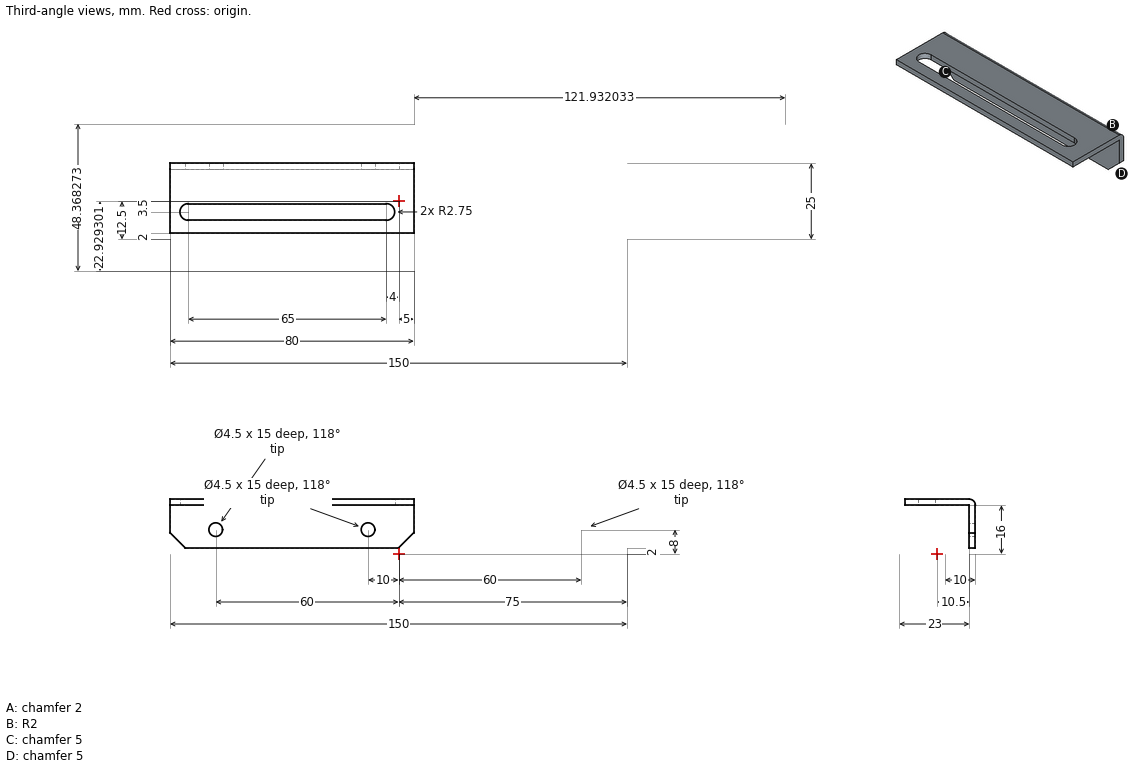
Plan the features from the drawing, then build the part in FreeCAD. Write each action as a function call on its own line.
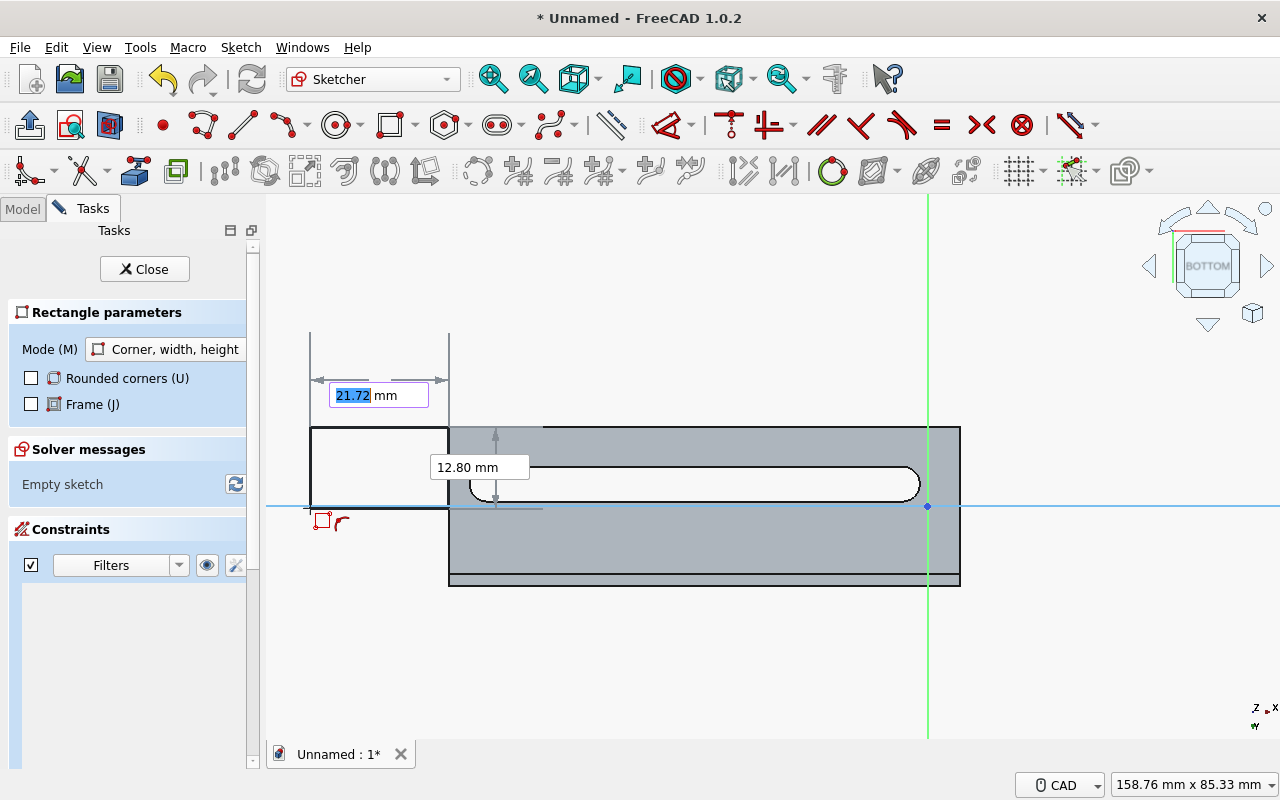
click(960, 439)
key(Escape)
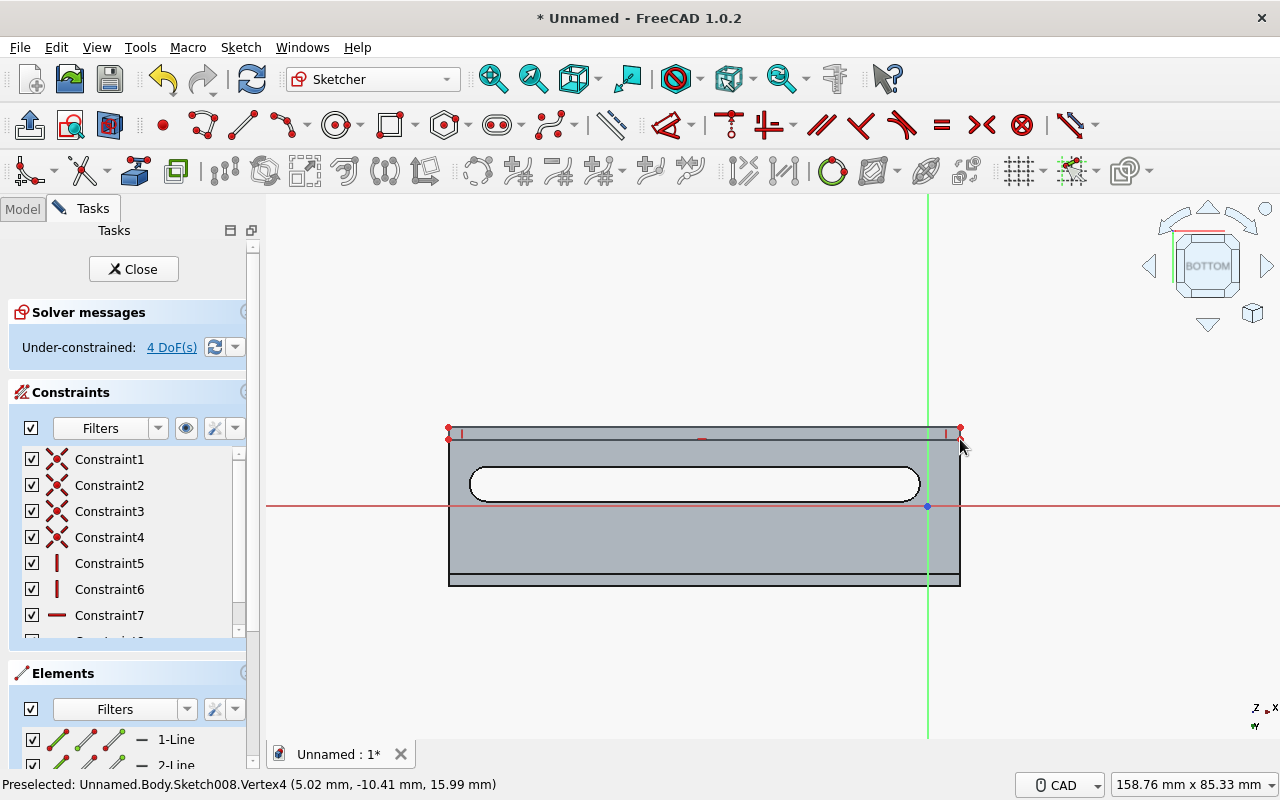
click(666, 126)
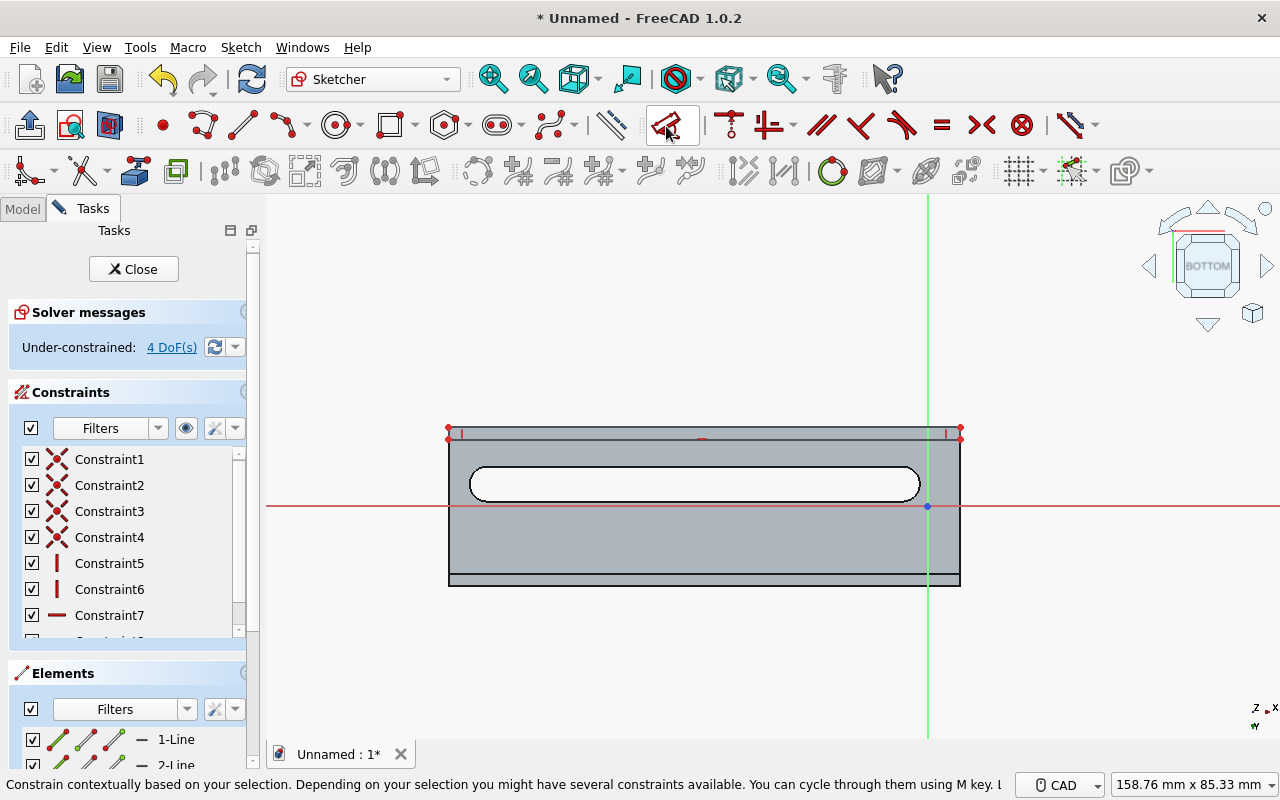
scroll(449, 434, up, 6)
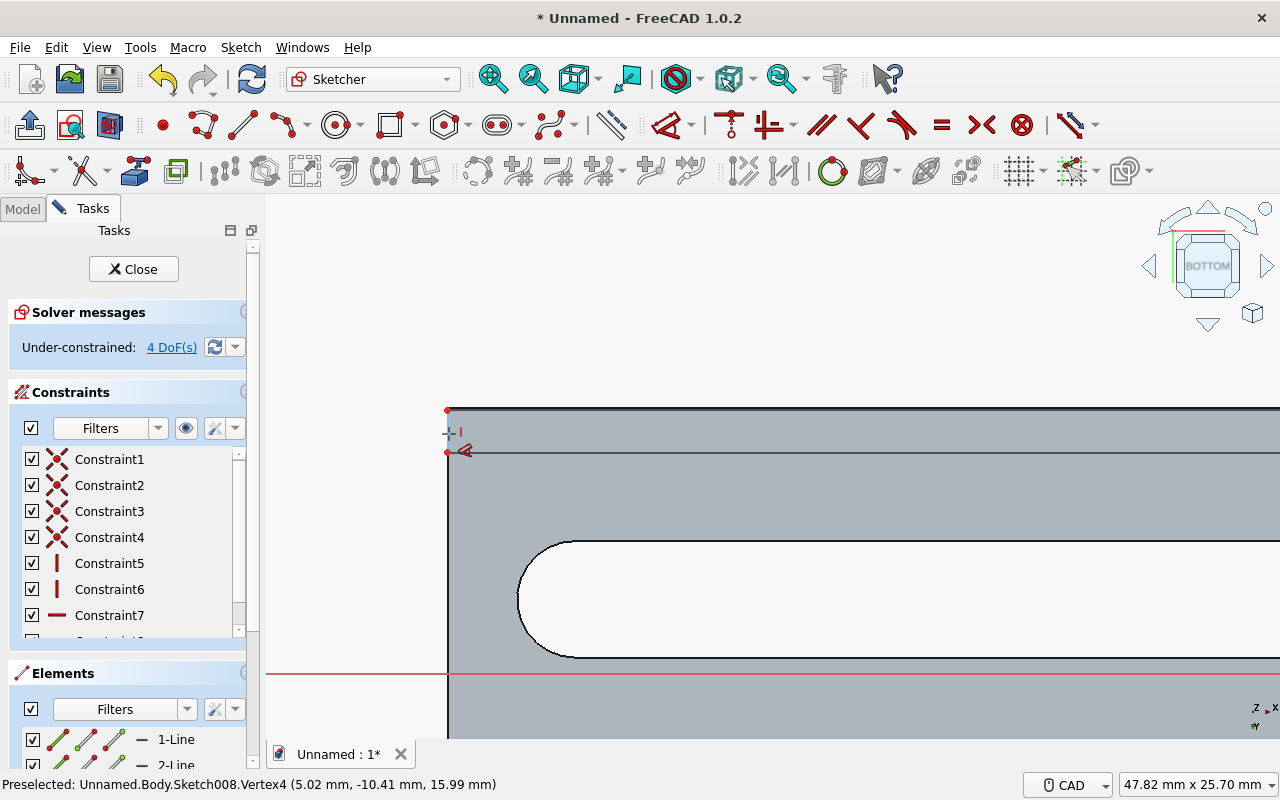
click(448, 431)
click(414, 431)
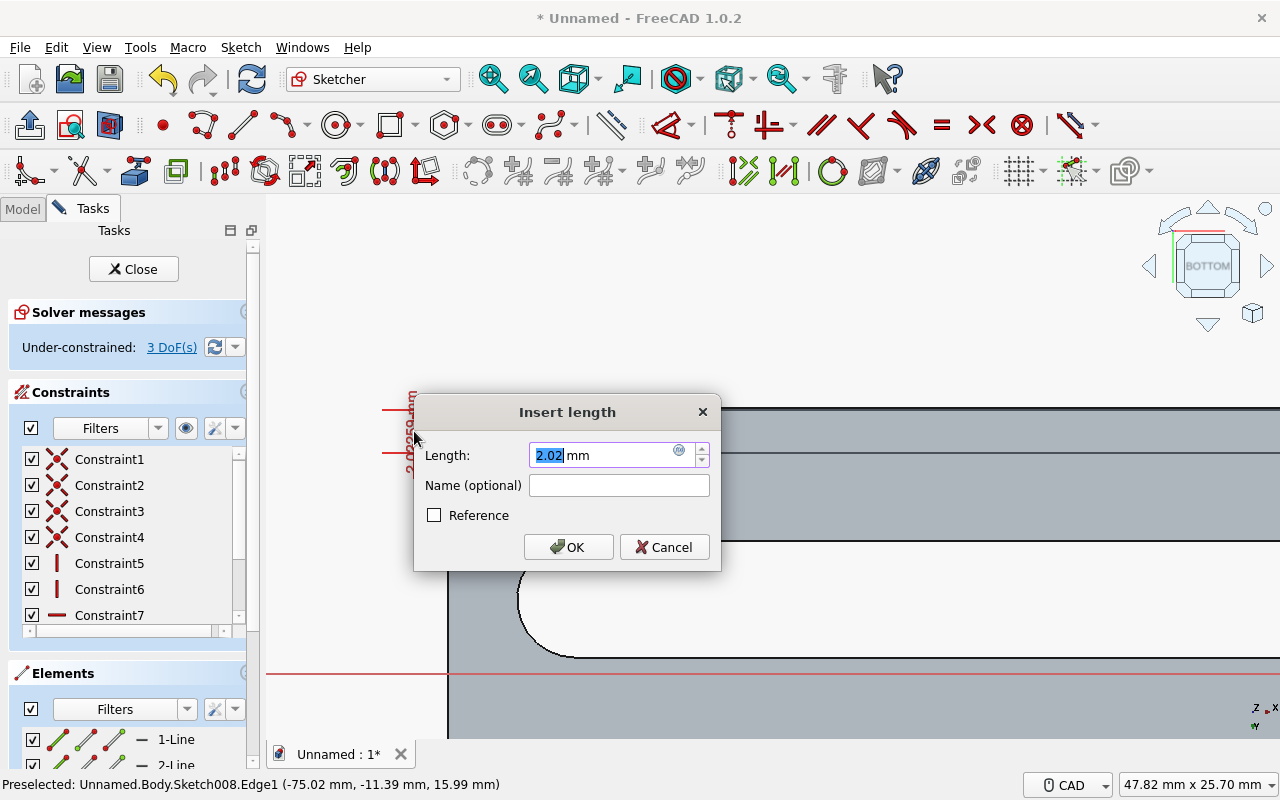
text(2)
key(Return)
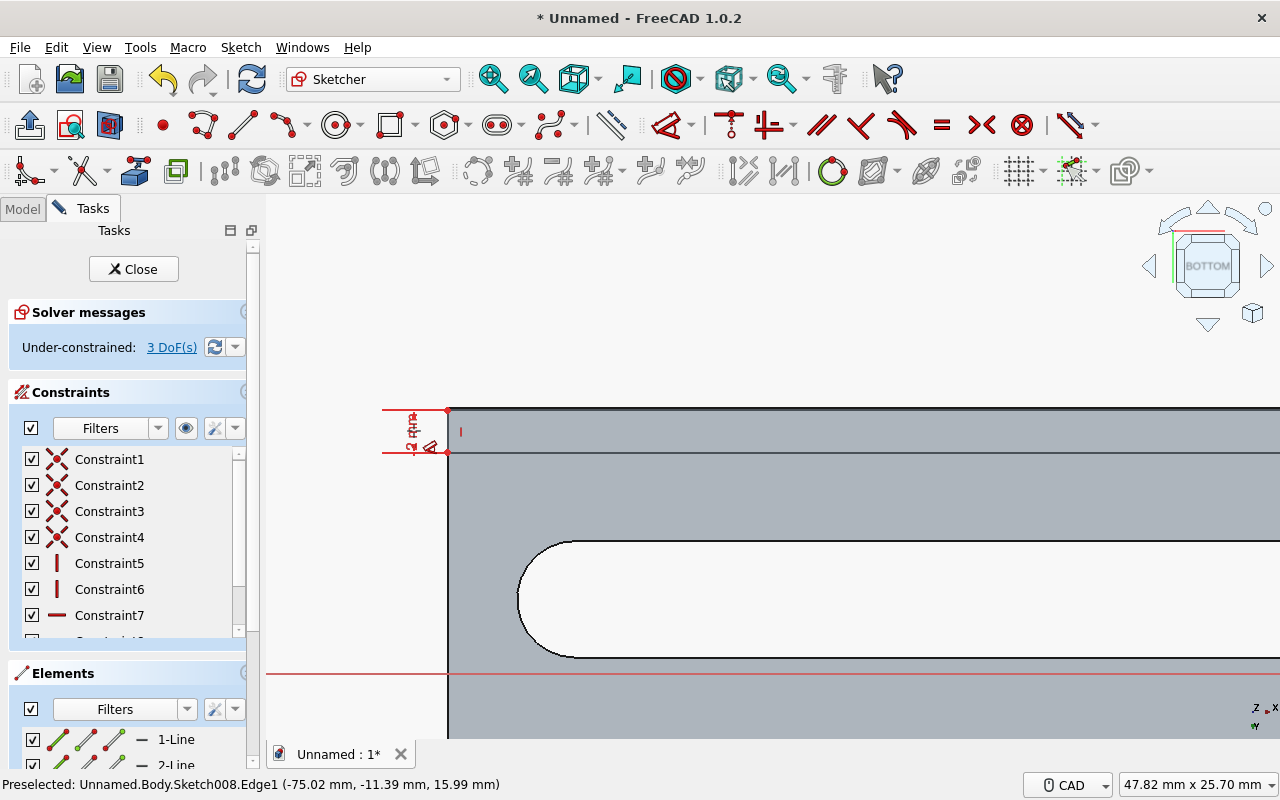
click(957, 453)
click(781, 487)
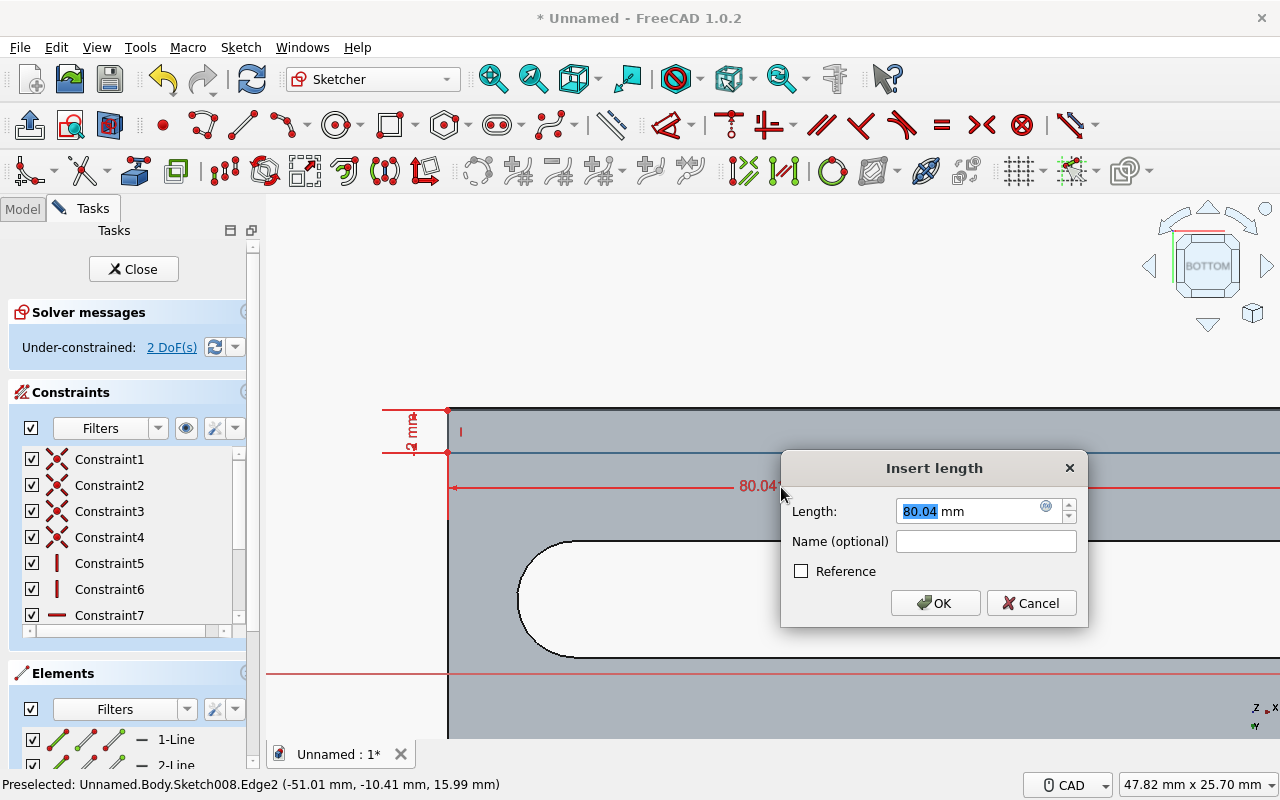
text(80)
key(Return)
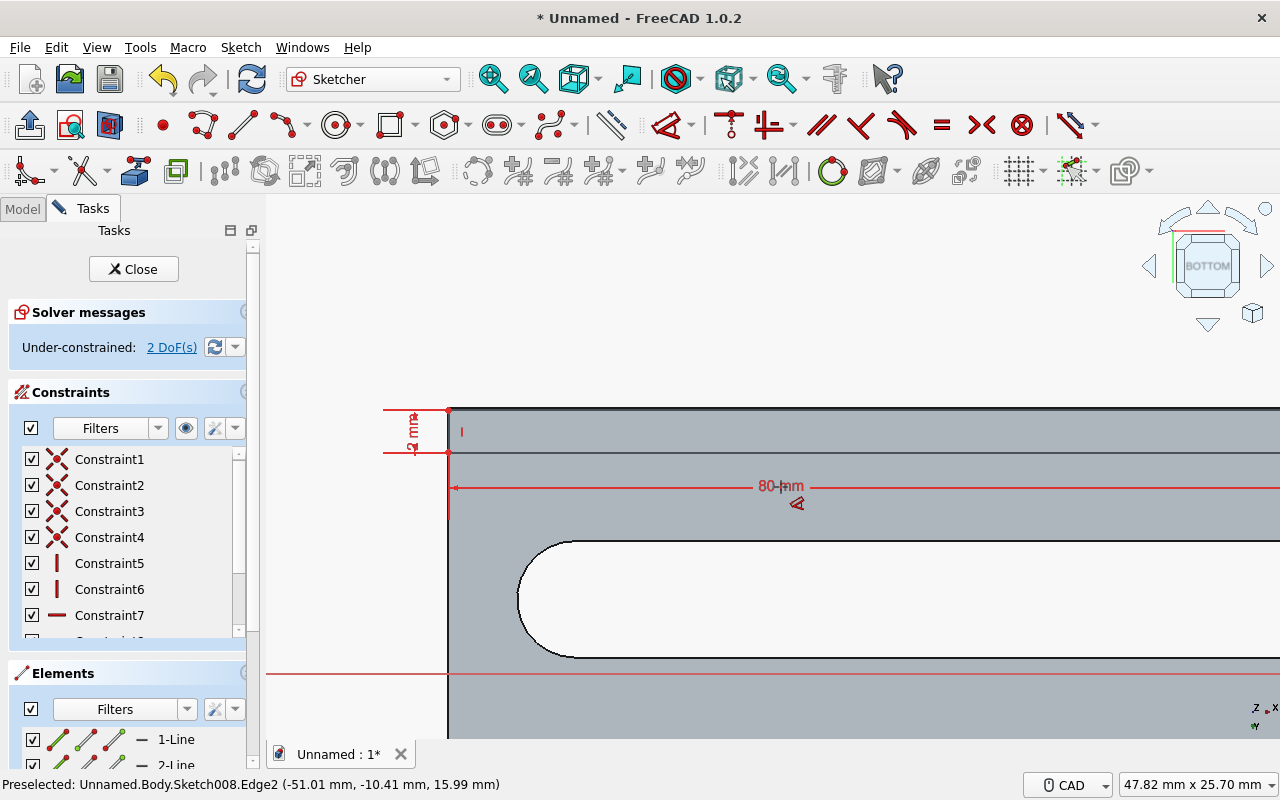
scroll(360, 423, down, 5)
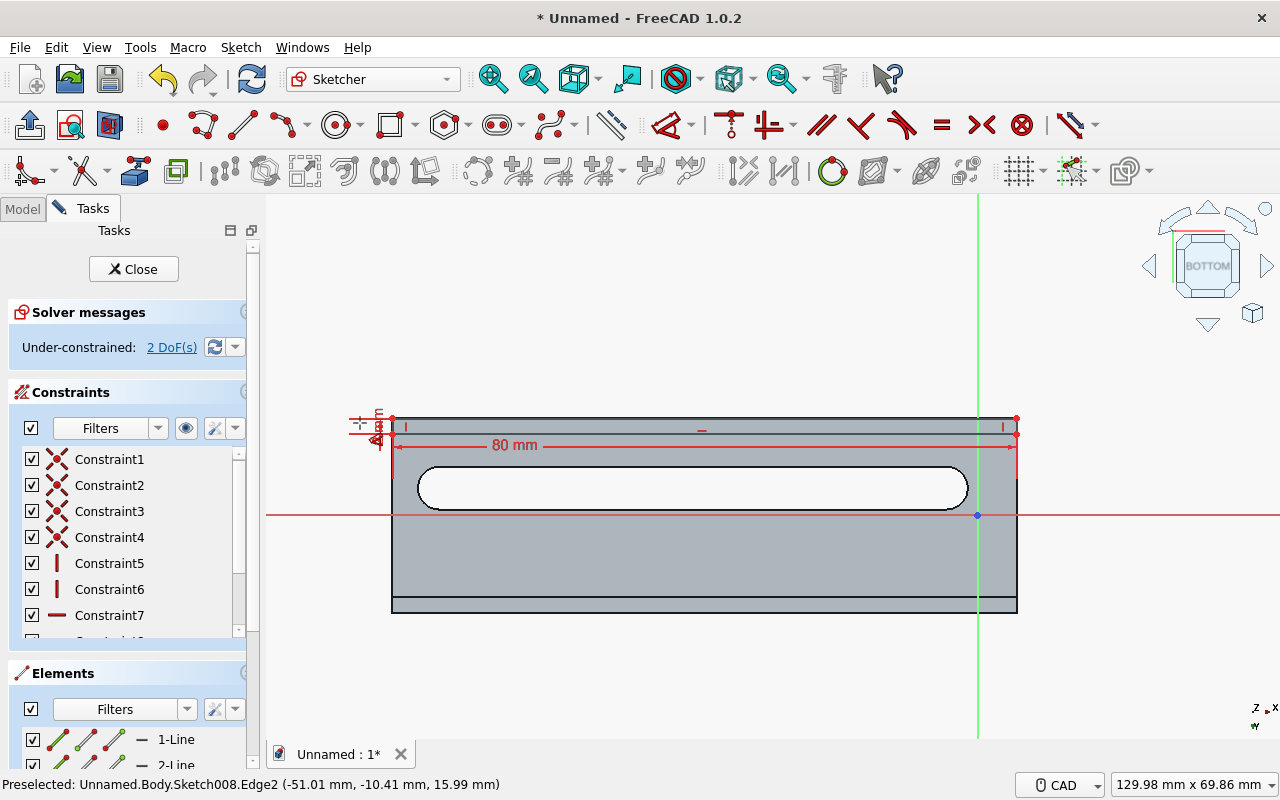
click(1017, 434)
click(997, 549)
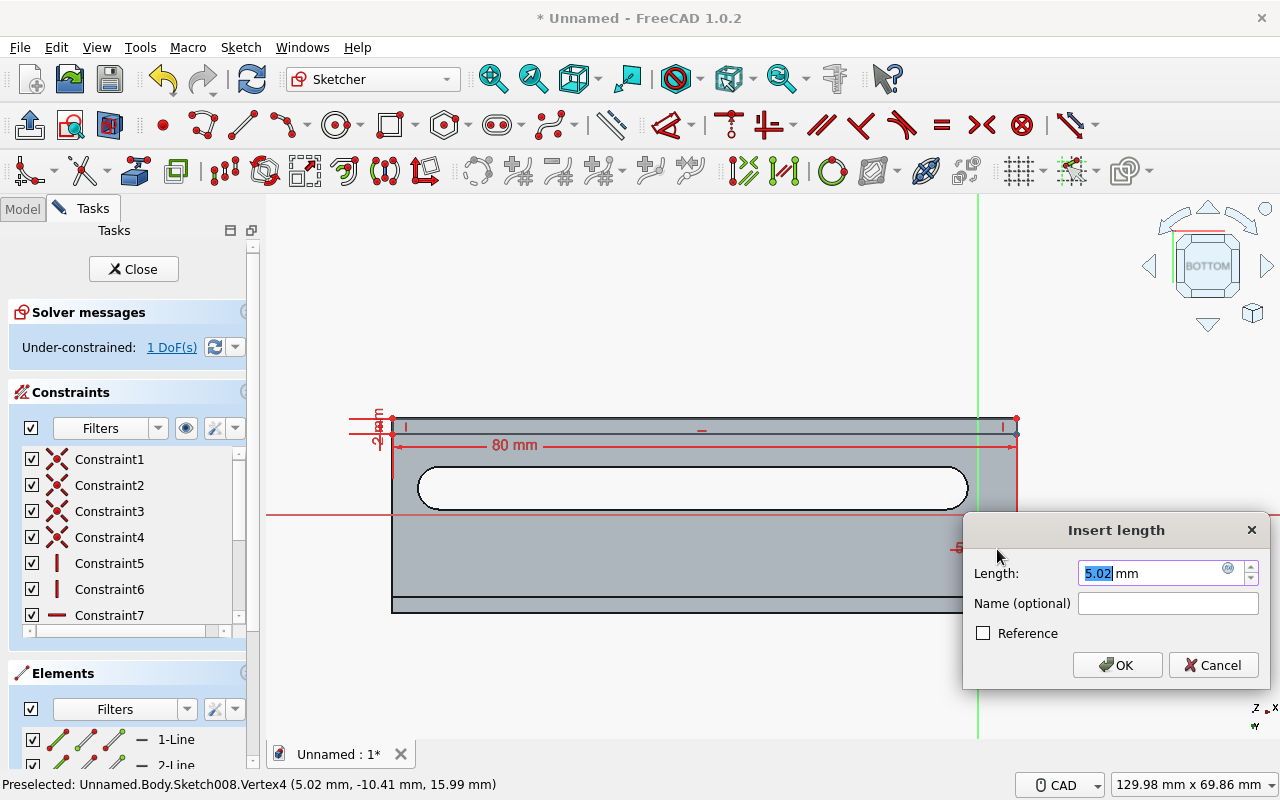
text(5)
key(Return)